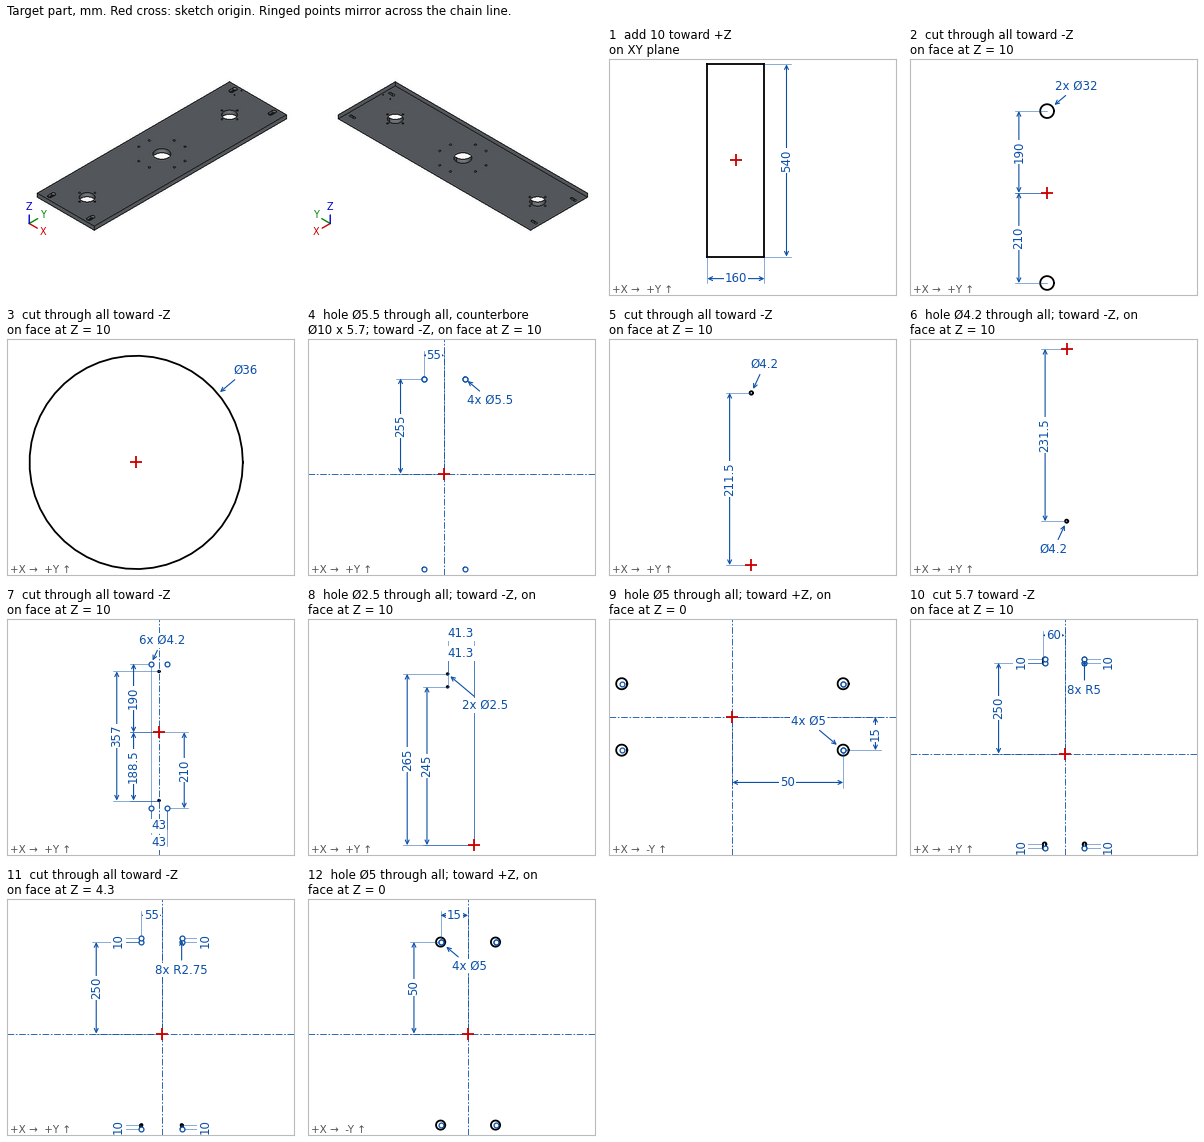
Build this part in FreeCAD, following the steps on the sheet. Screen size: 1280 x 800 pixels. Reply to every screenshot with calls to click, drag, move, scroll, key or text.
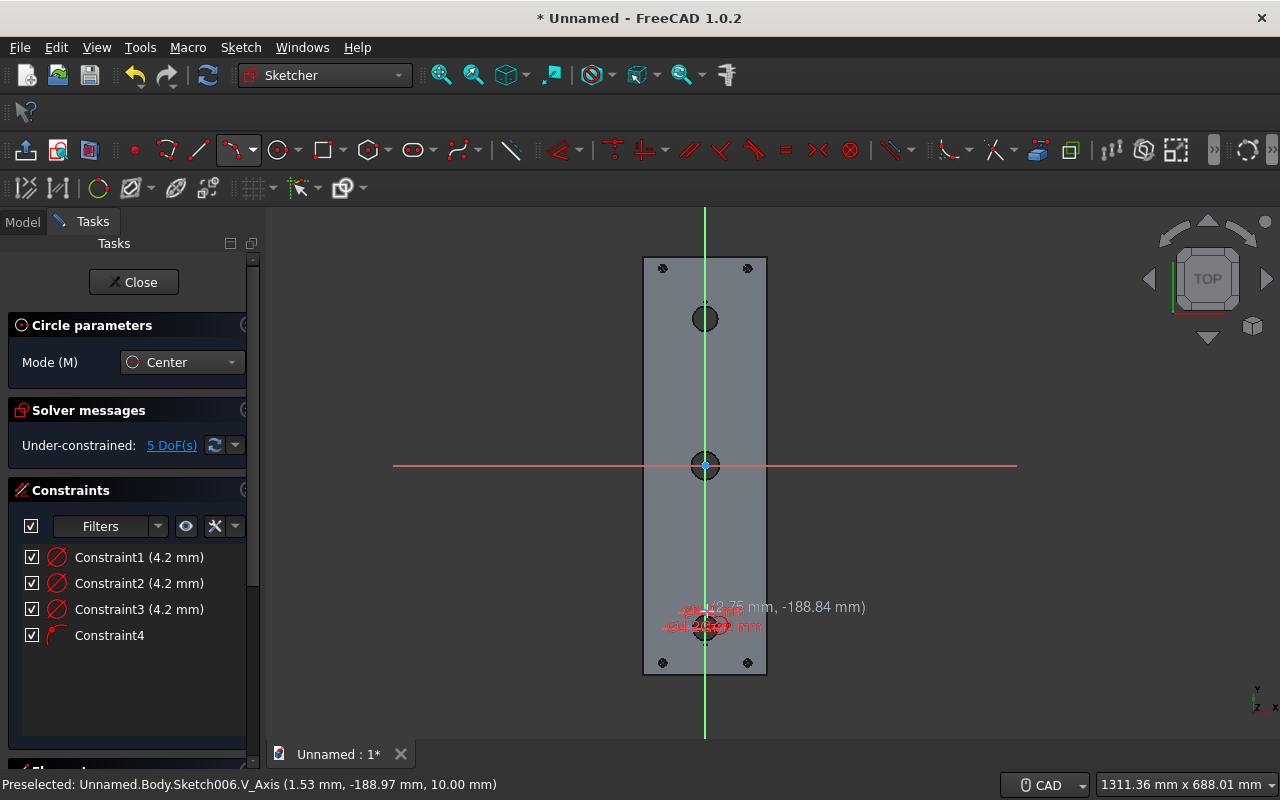
scroll(689, 319, up, 14)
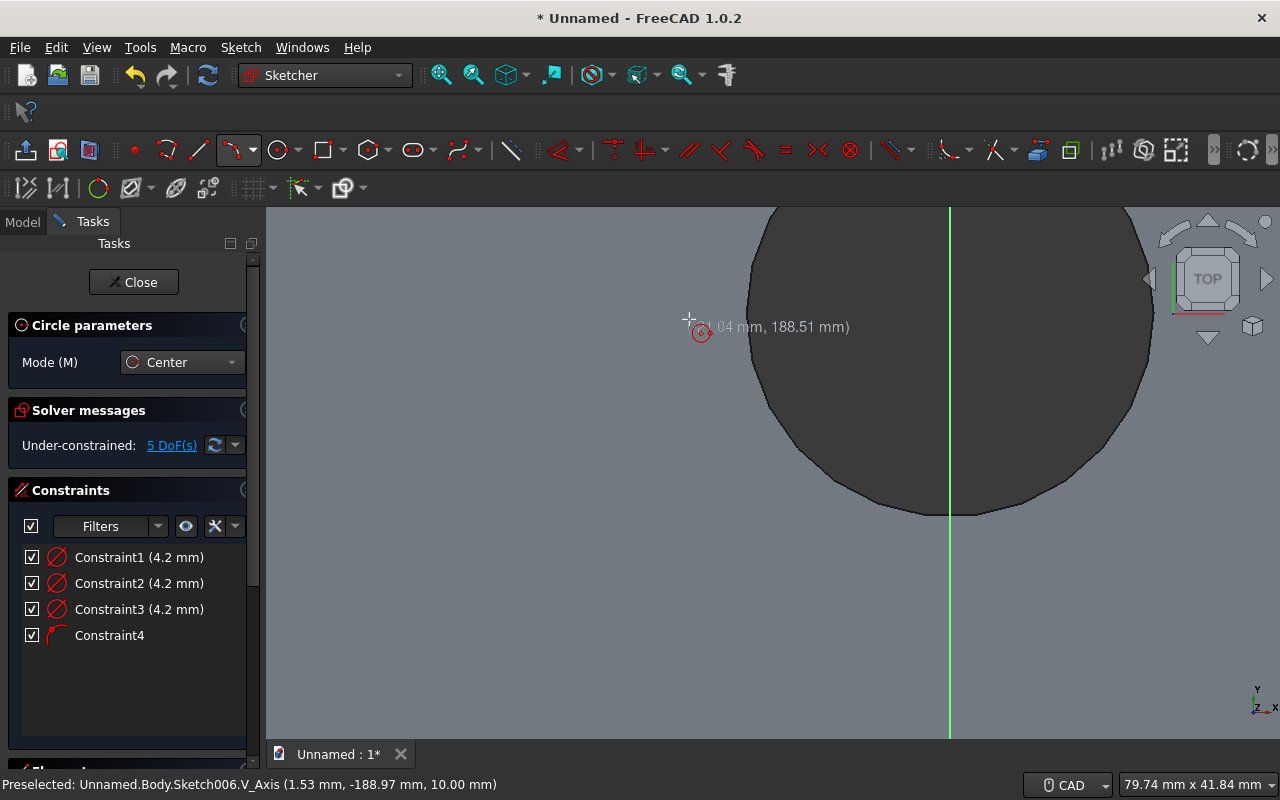
scroll(689, 319, down, 14)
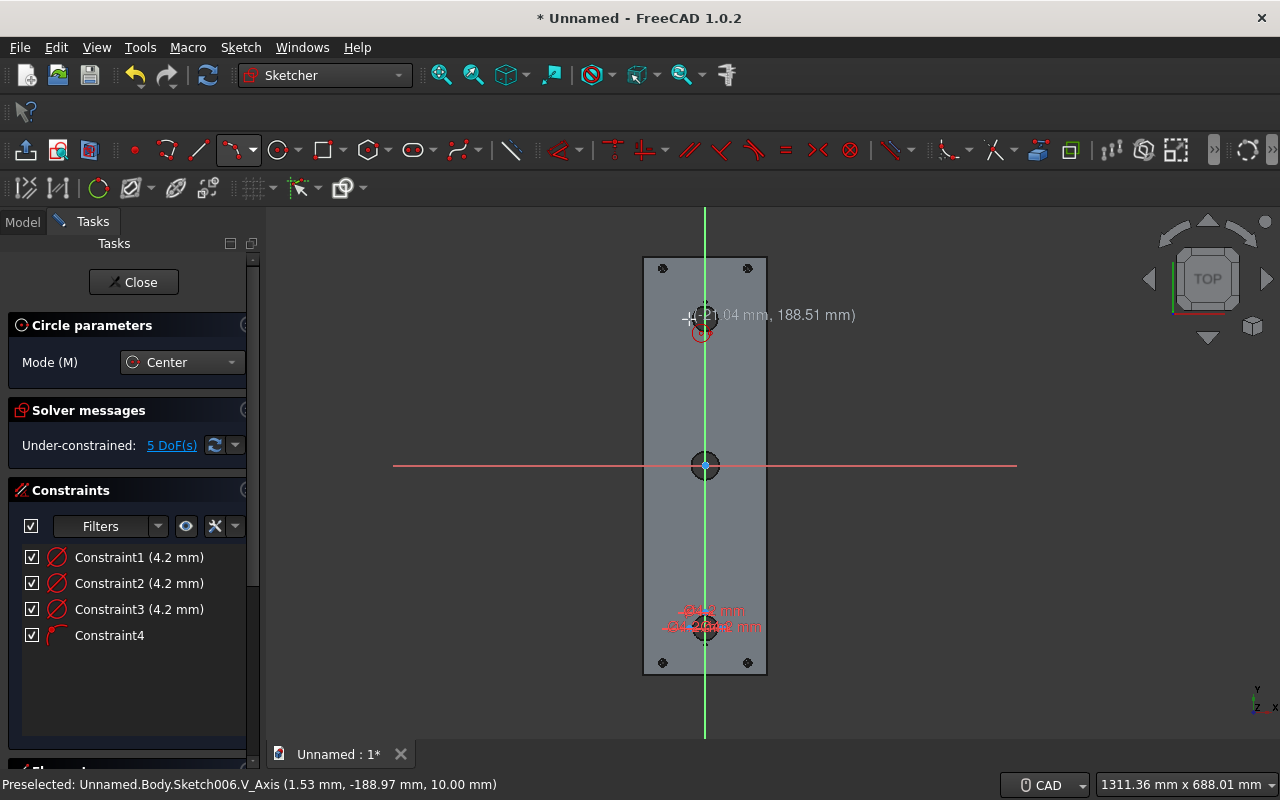
click(689, 319)
move(690, 318)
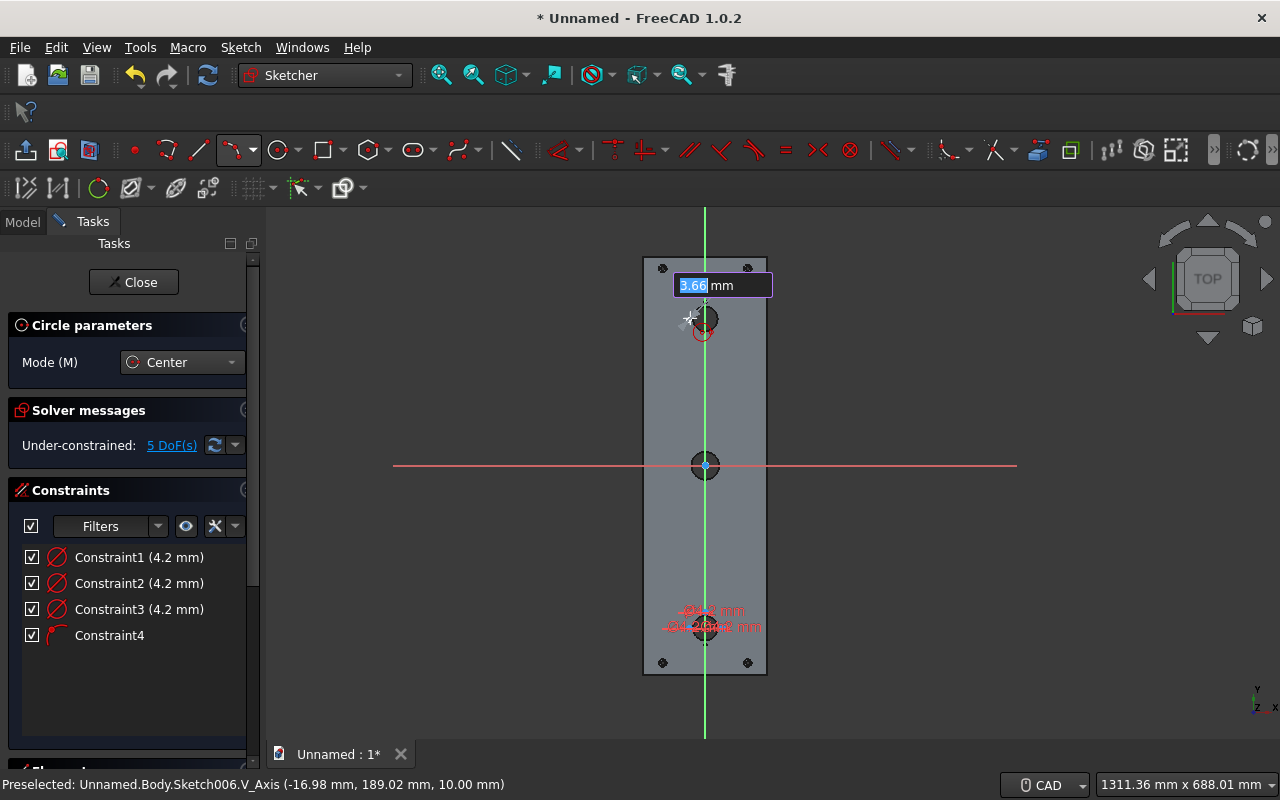
text(4.2)
key(Return)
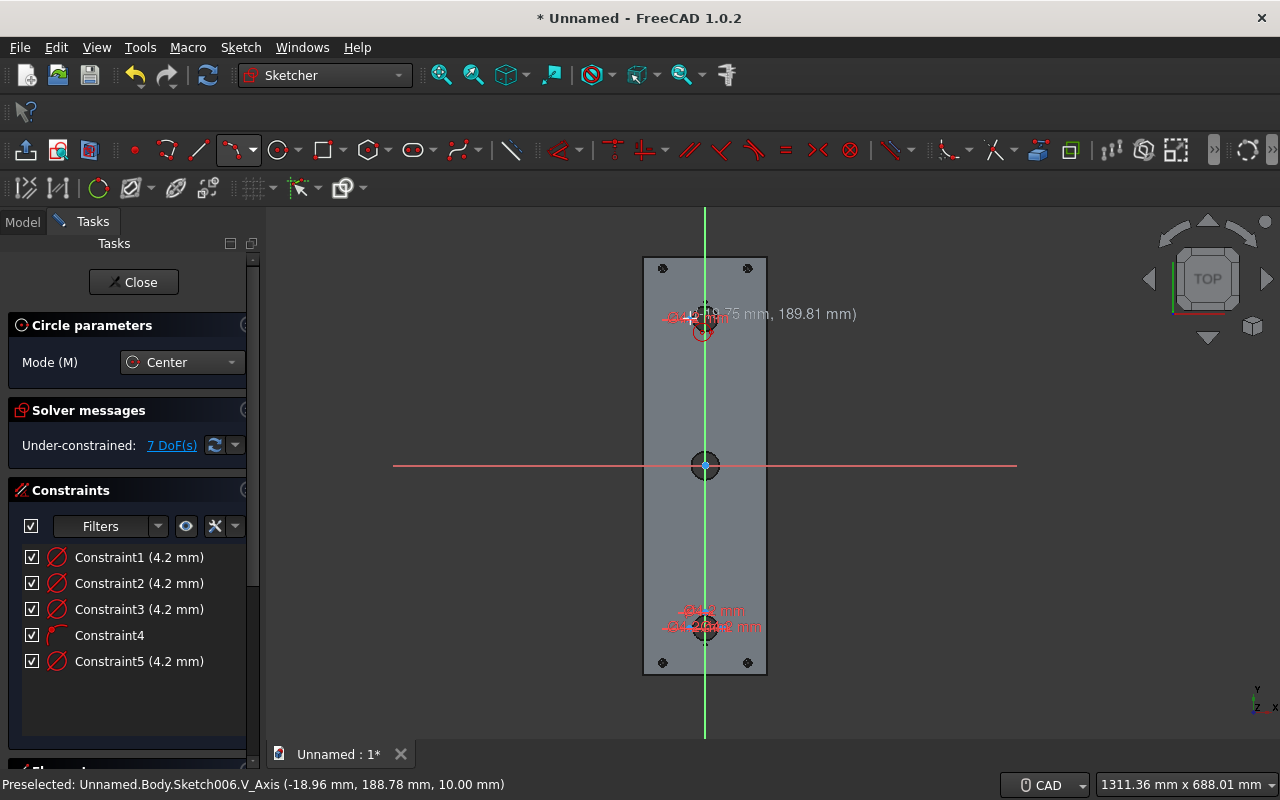
scroll(722, 319, up, 14)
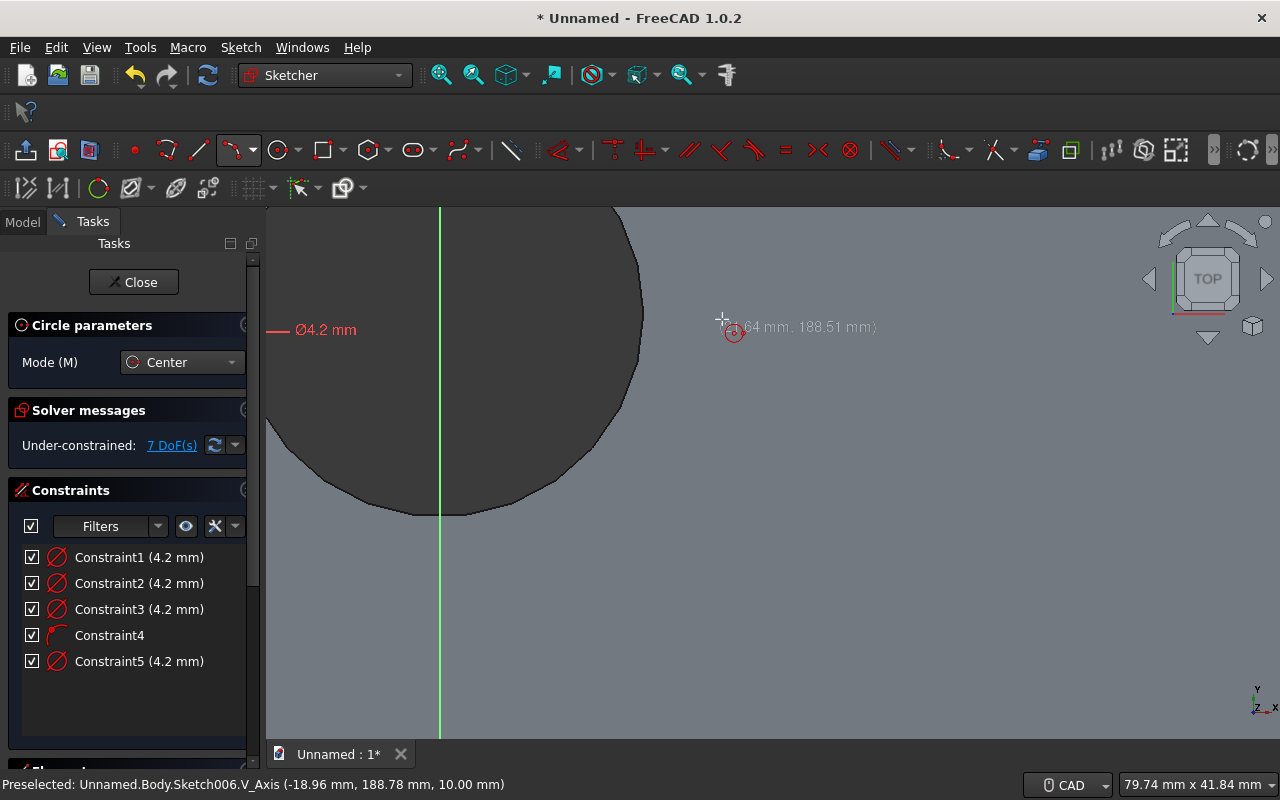
scroll(722, 319, down, 14)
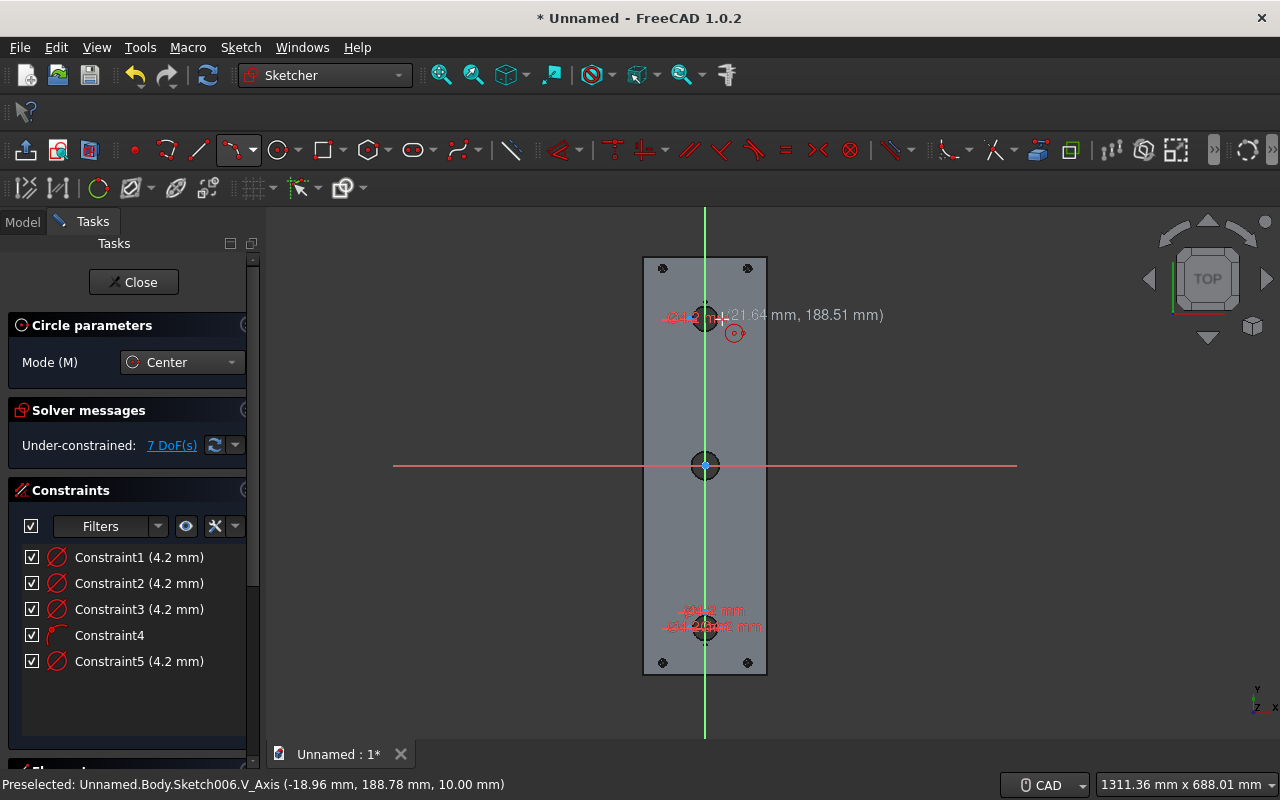
click(722, 319)
move(723, 318)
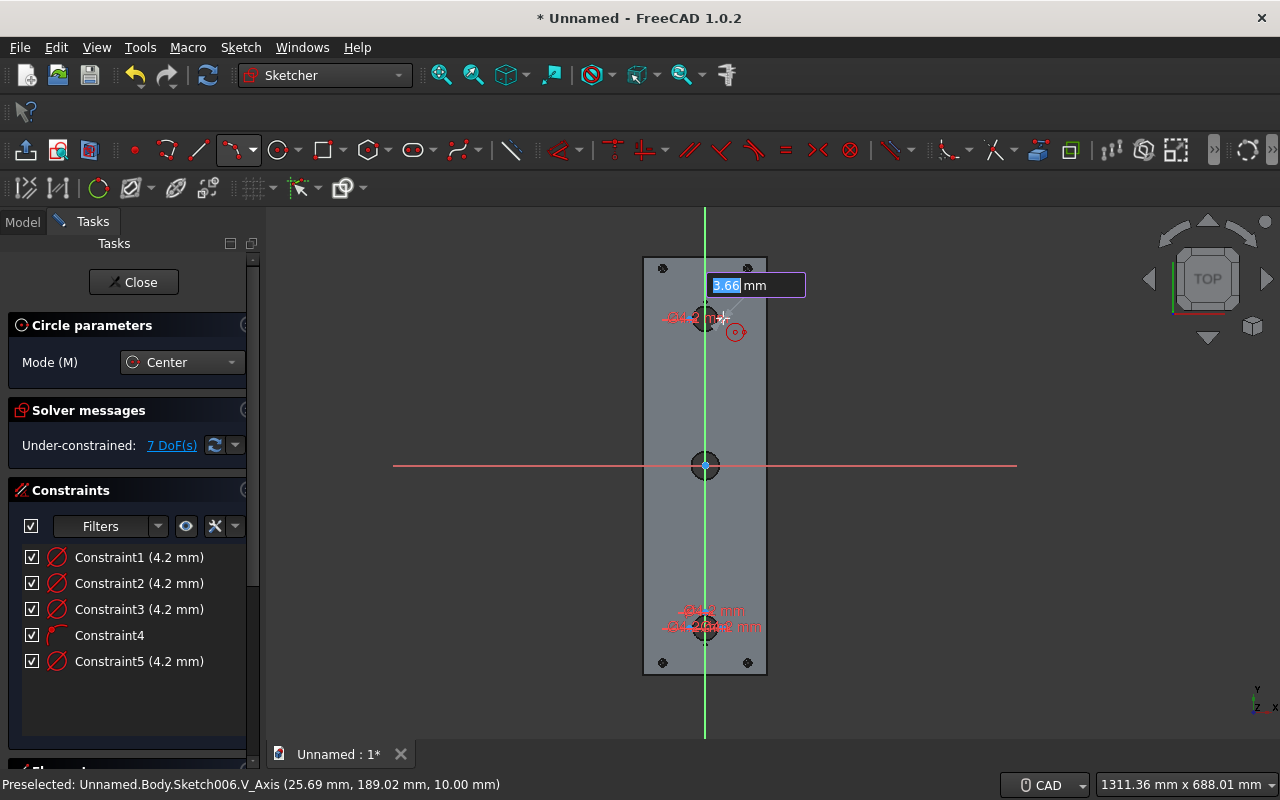
text(4.2)
key(Return)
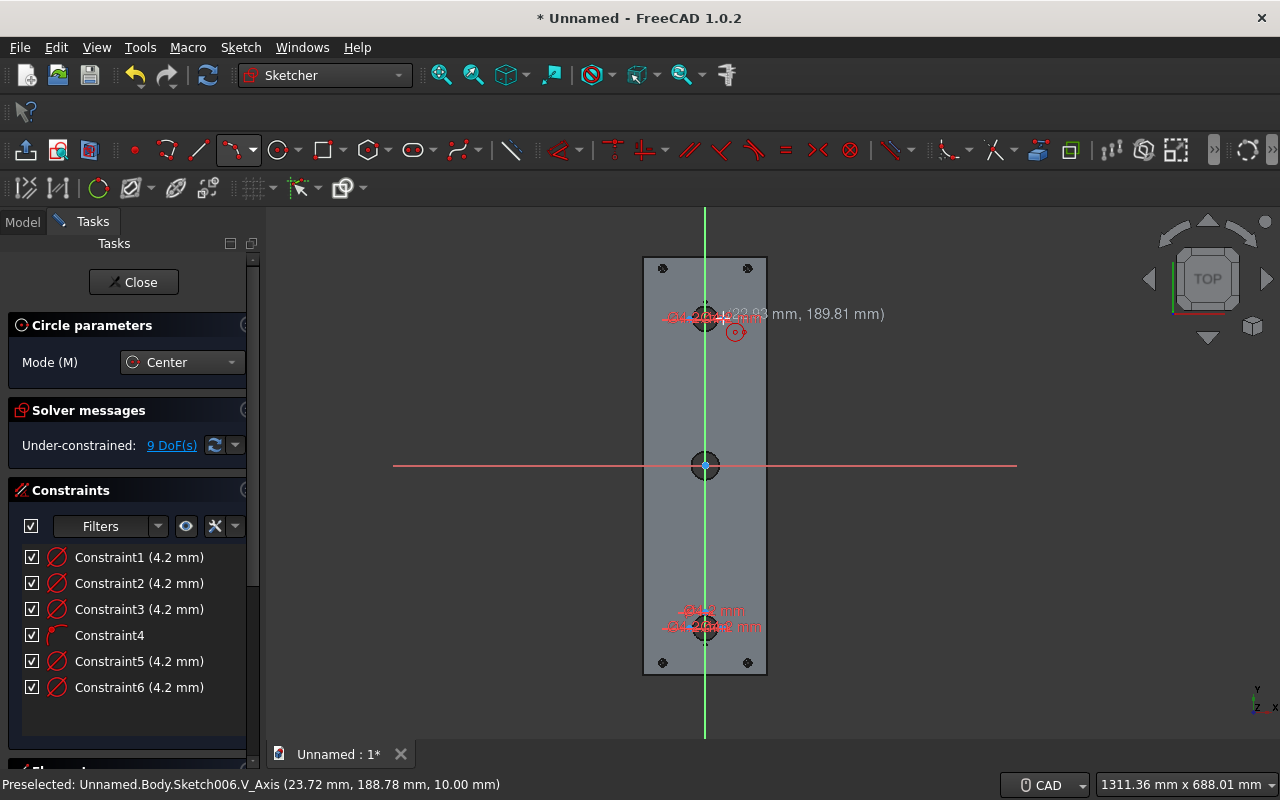
scroll(705, 335, up, 14)